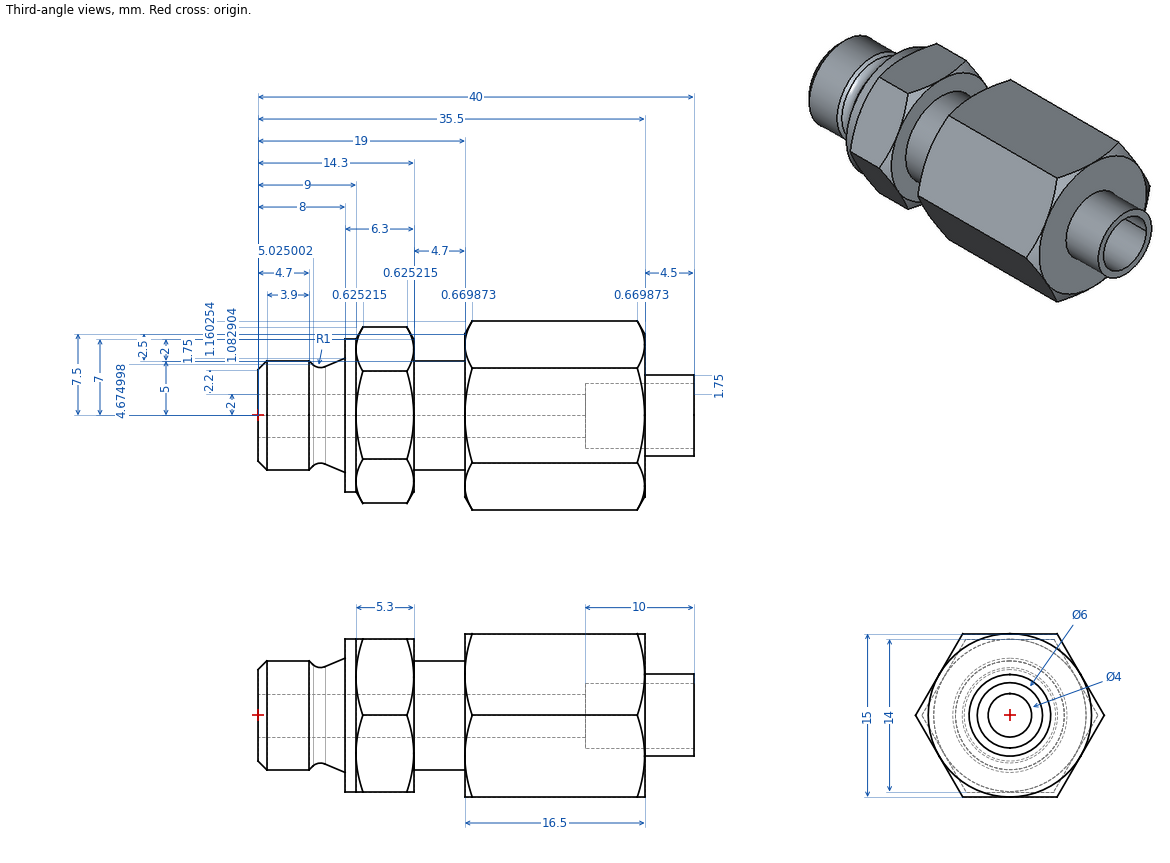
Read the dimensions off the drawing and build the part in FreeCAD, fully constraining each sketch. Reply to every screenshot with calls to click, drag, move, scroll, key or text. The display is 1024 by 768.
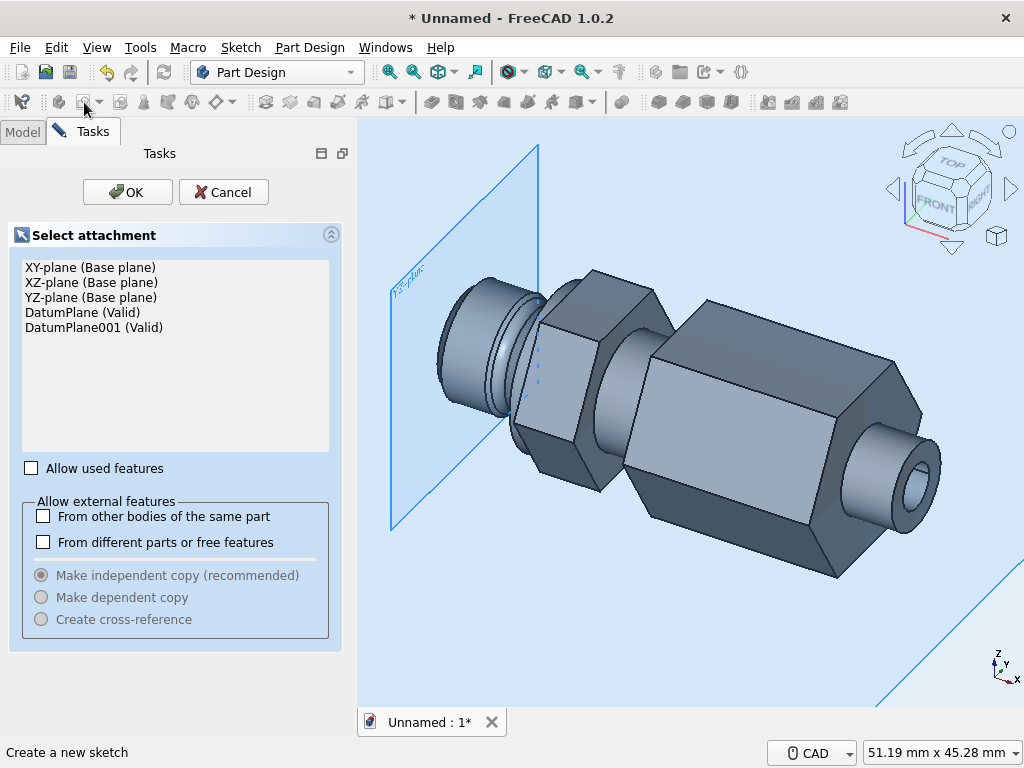
click(82, 268)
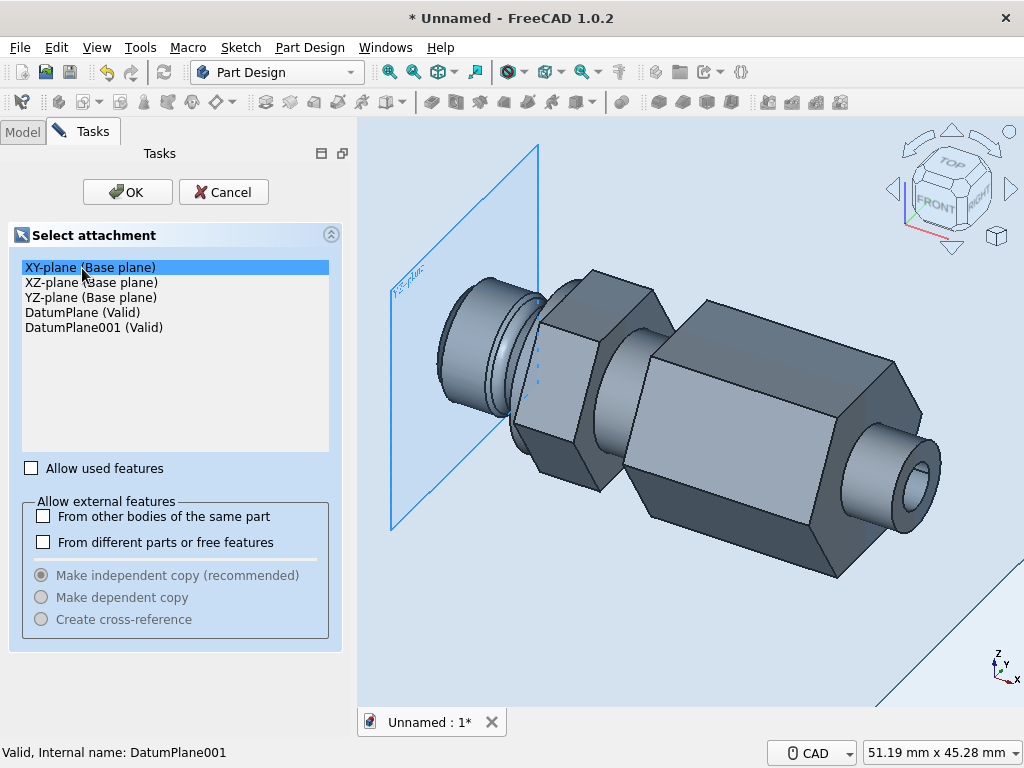
click(128, 192)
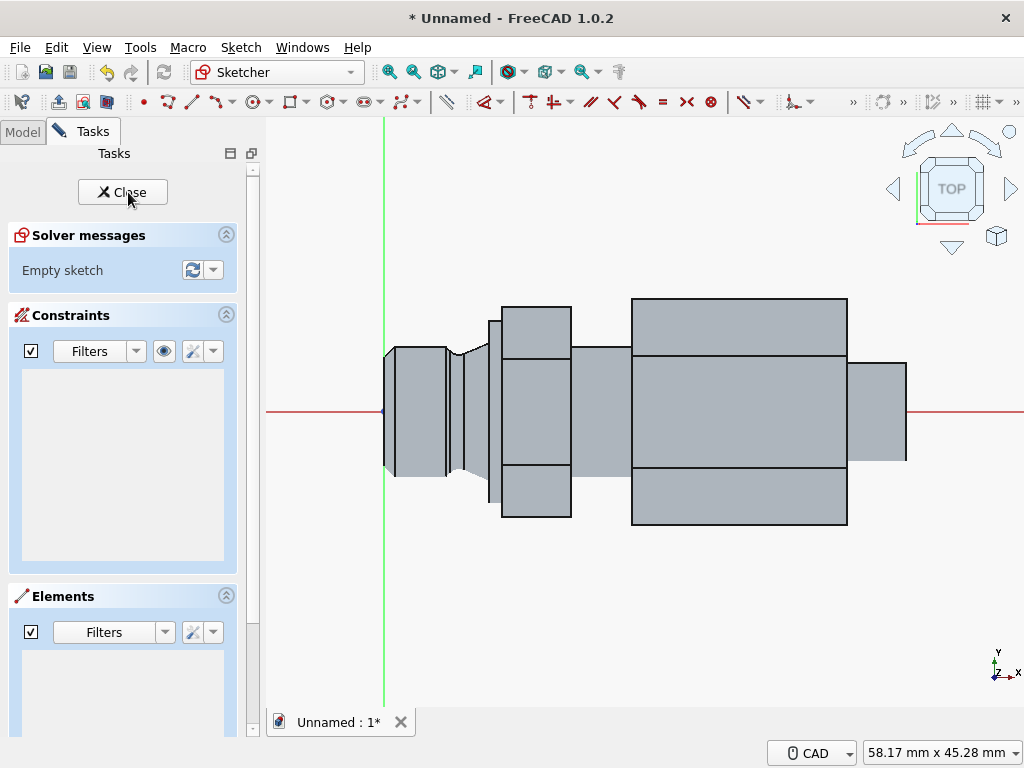
click(108, 102)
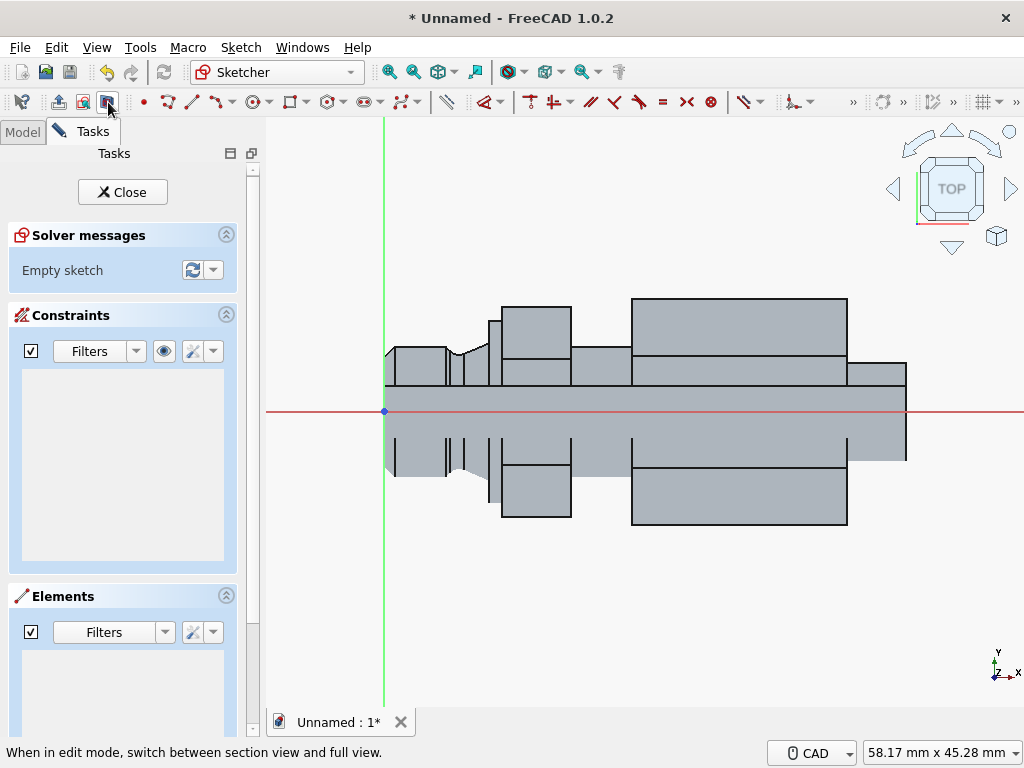
scroll(400, 667, down, 1)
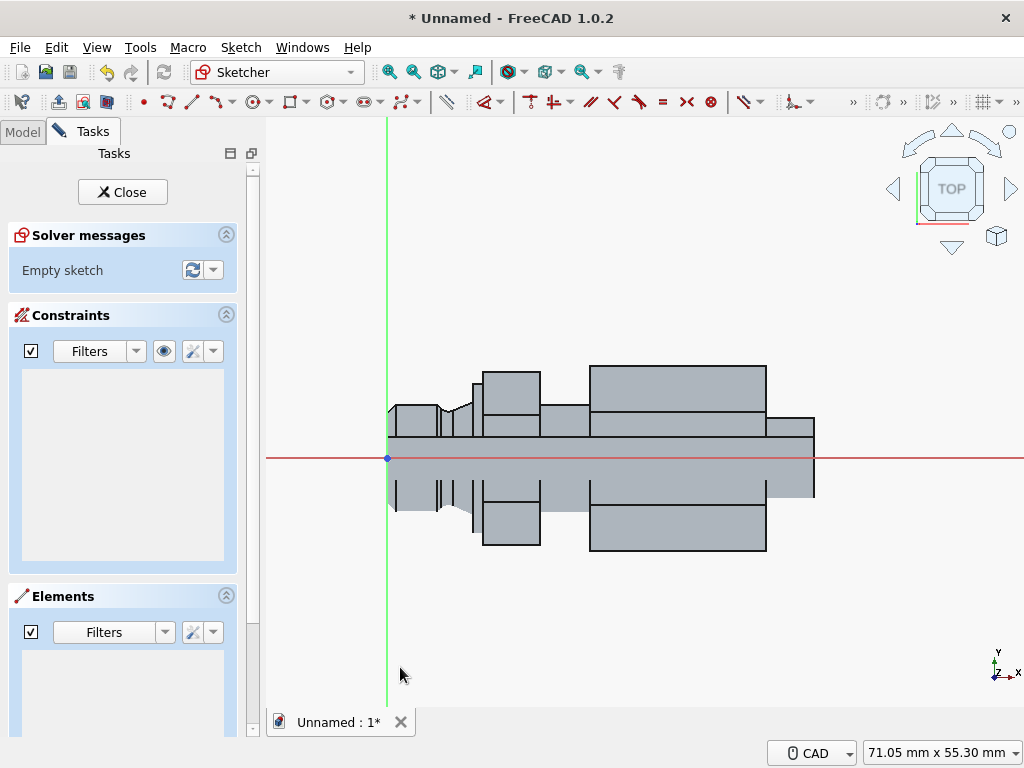
key(g)
key(m)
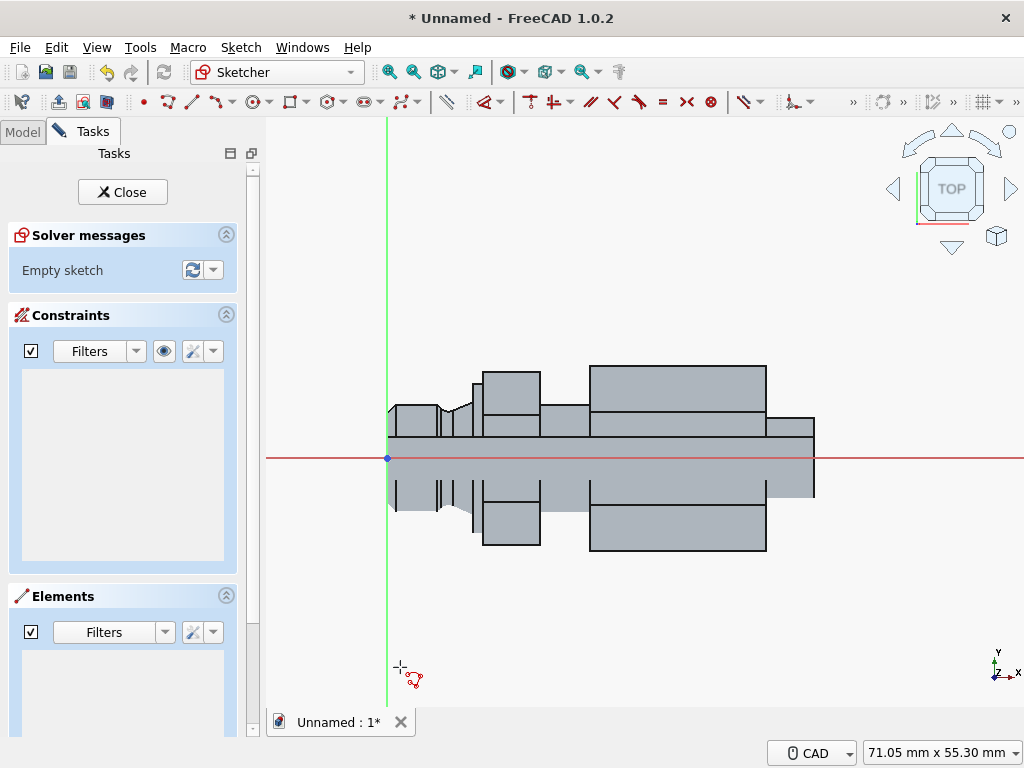
click(483, 384)
click(490, 372)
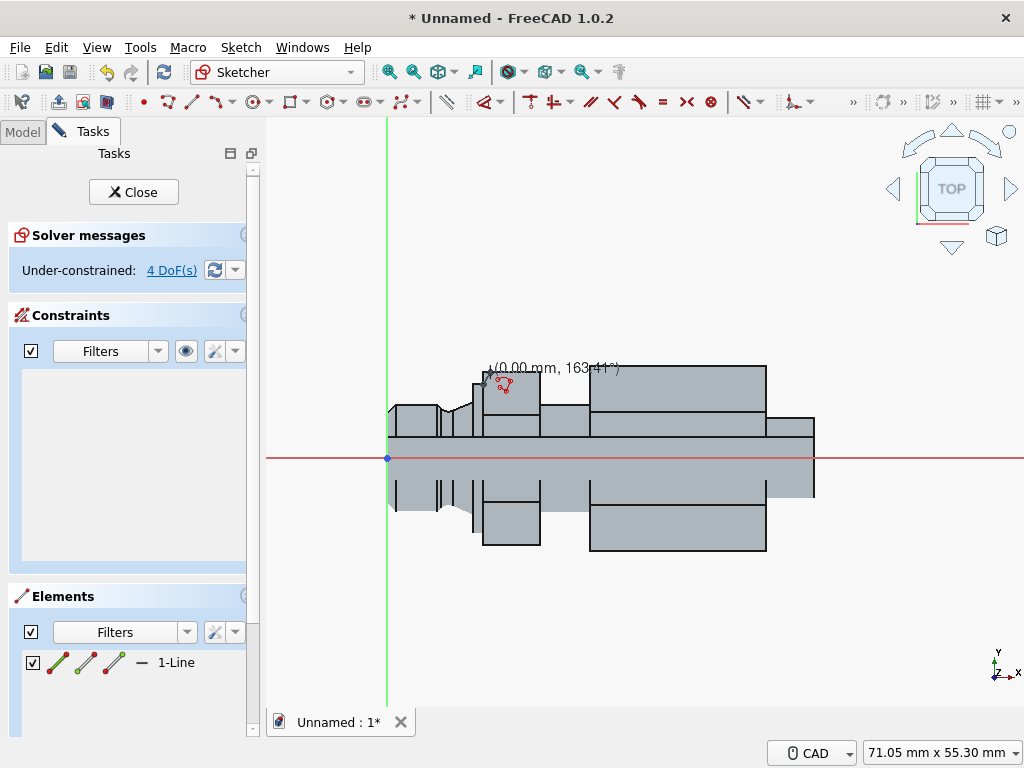
scroll(483, 372, up, 6)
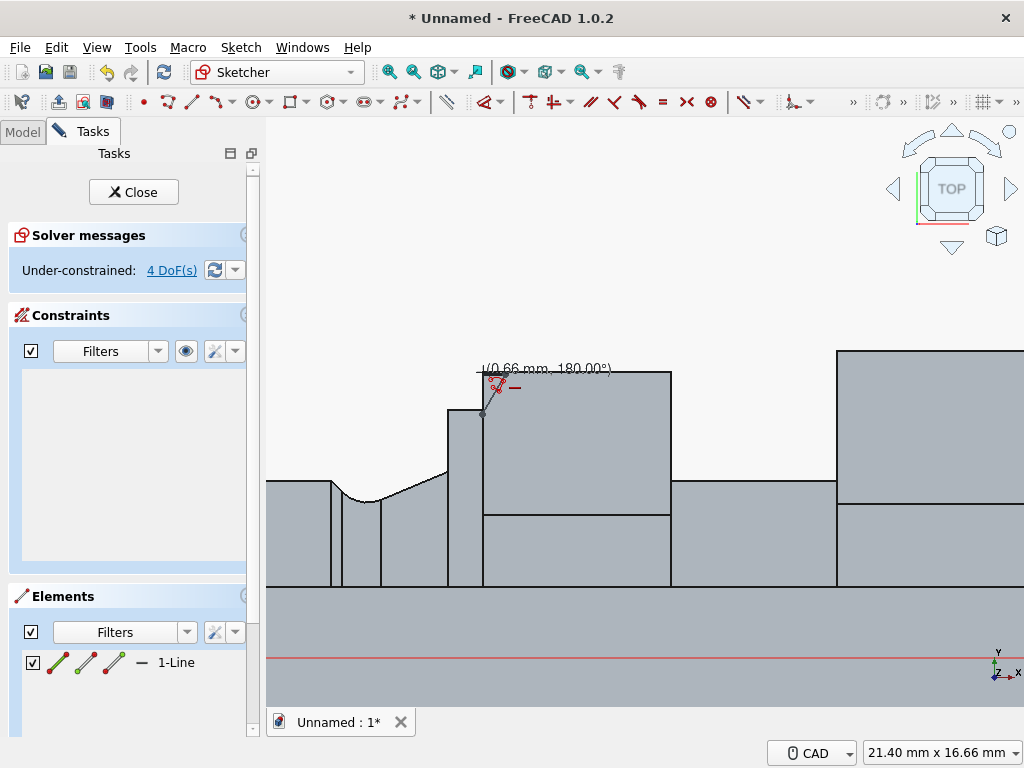
click(483, 371)
click(482, 414)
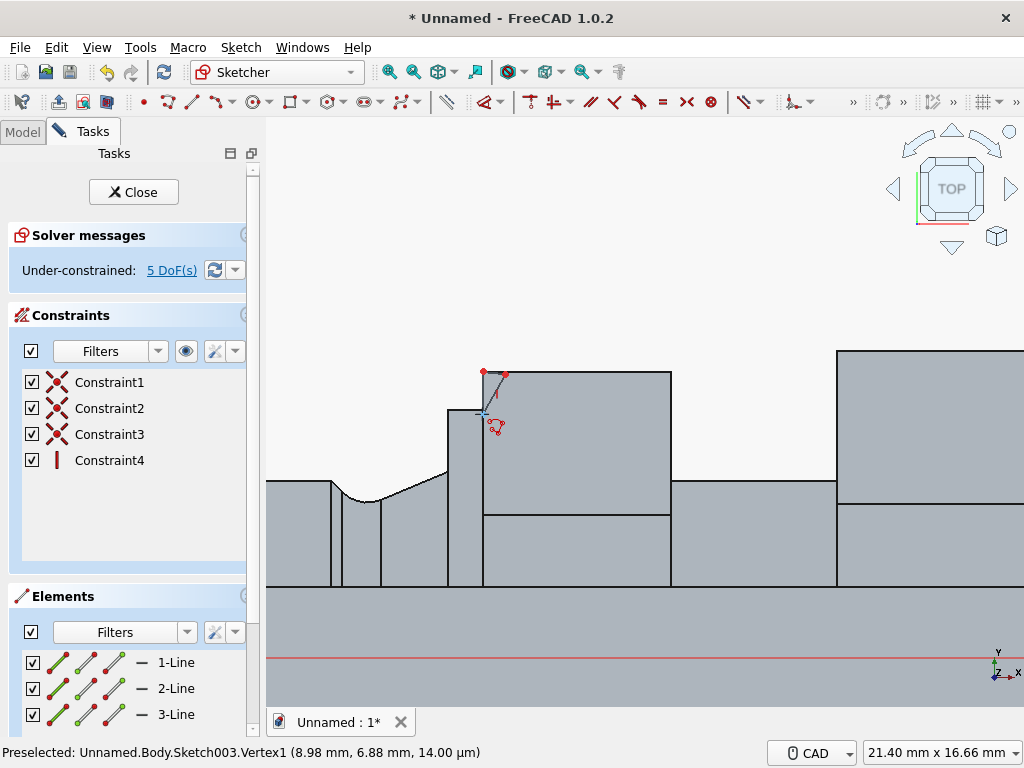
click(649, 372)
click(671, 410)
click(671, 372)
click(649, 373)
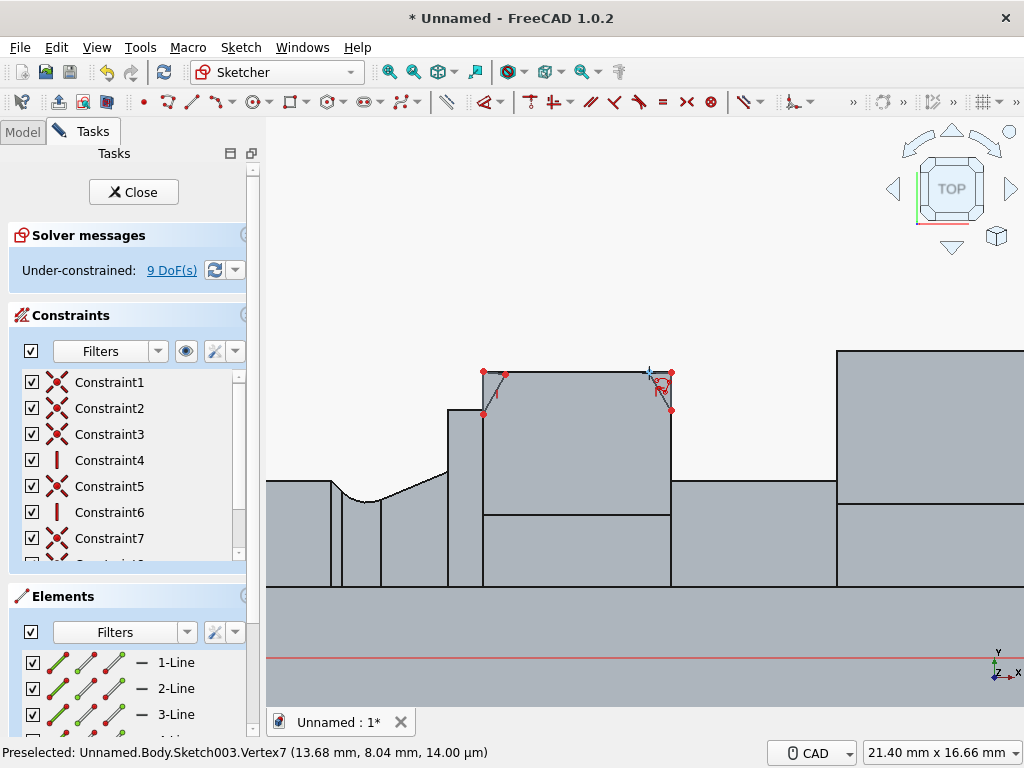
click(837, 392)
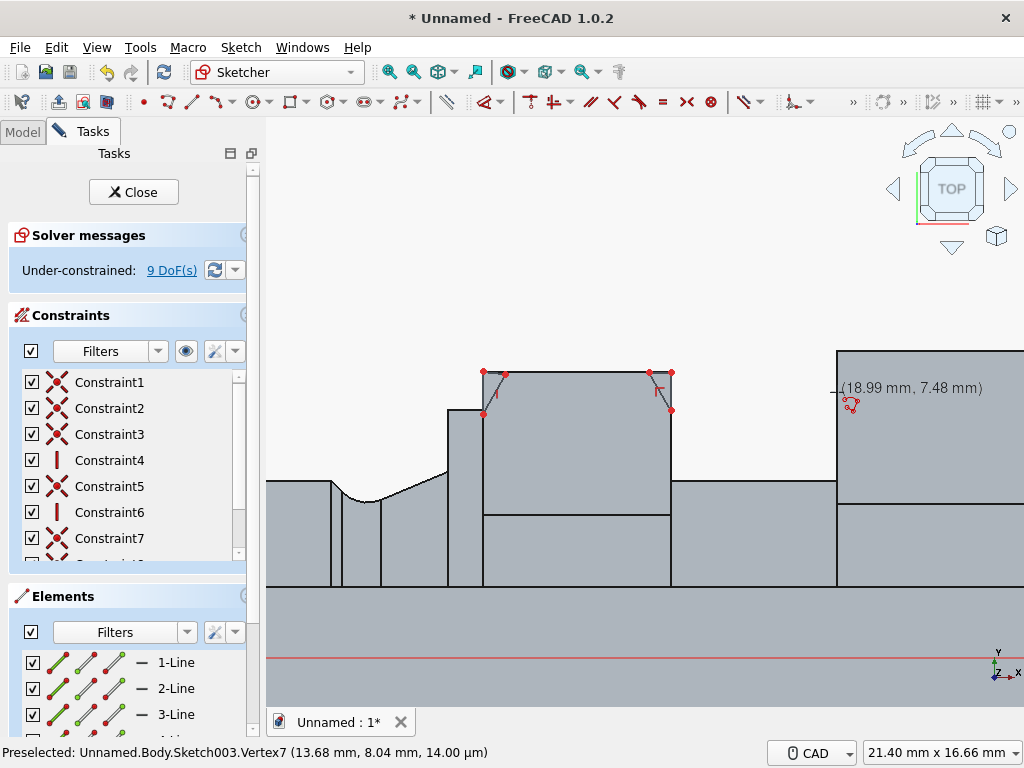
scroll(483, 372, down, 6)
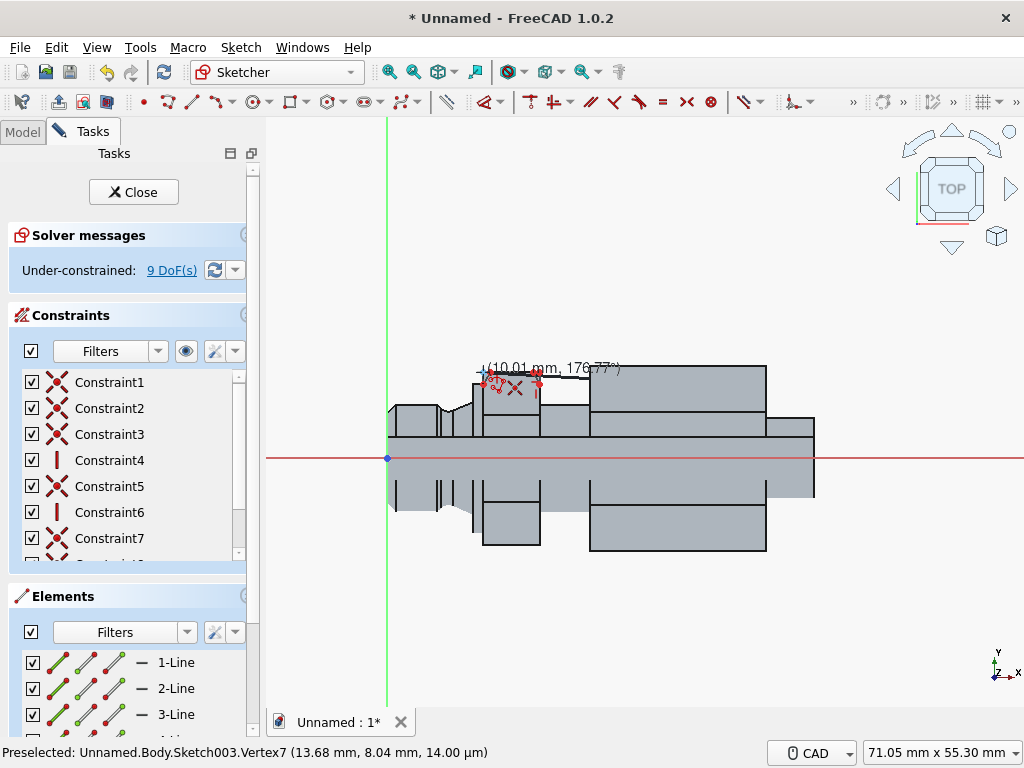
click(597, 366)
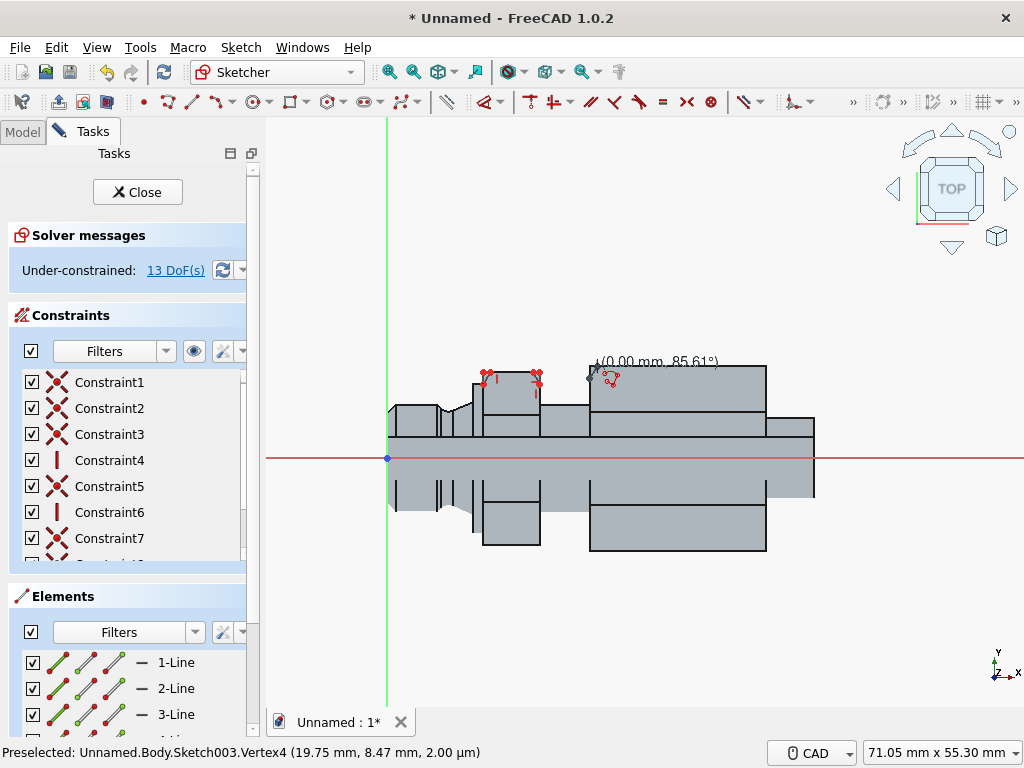
scroll(590, 366, up, 5)